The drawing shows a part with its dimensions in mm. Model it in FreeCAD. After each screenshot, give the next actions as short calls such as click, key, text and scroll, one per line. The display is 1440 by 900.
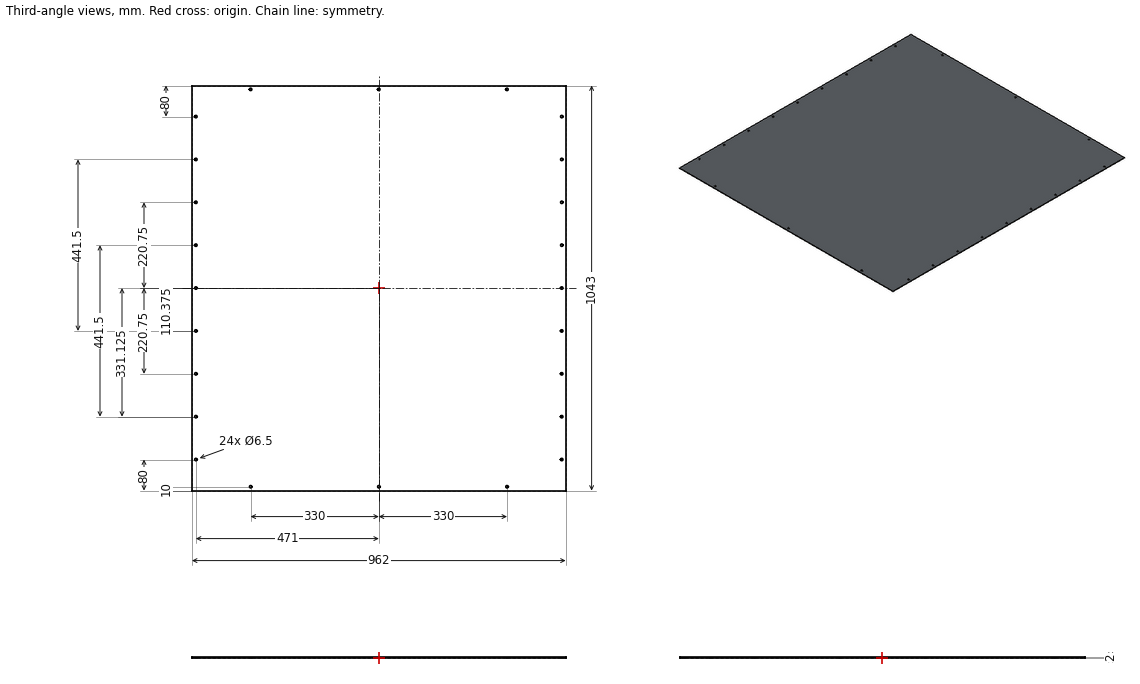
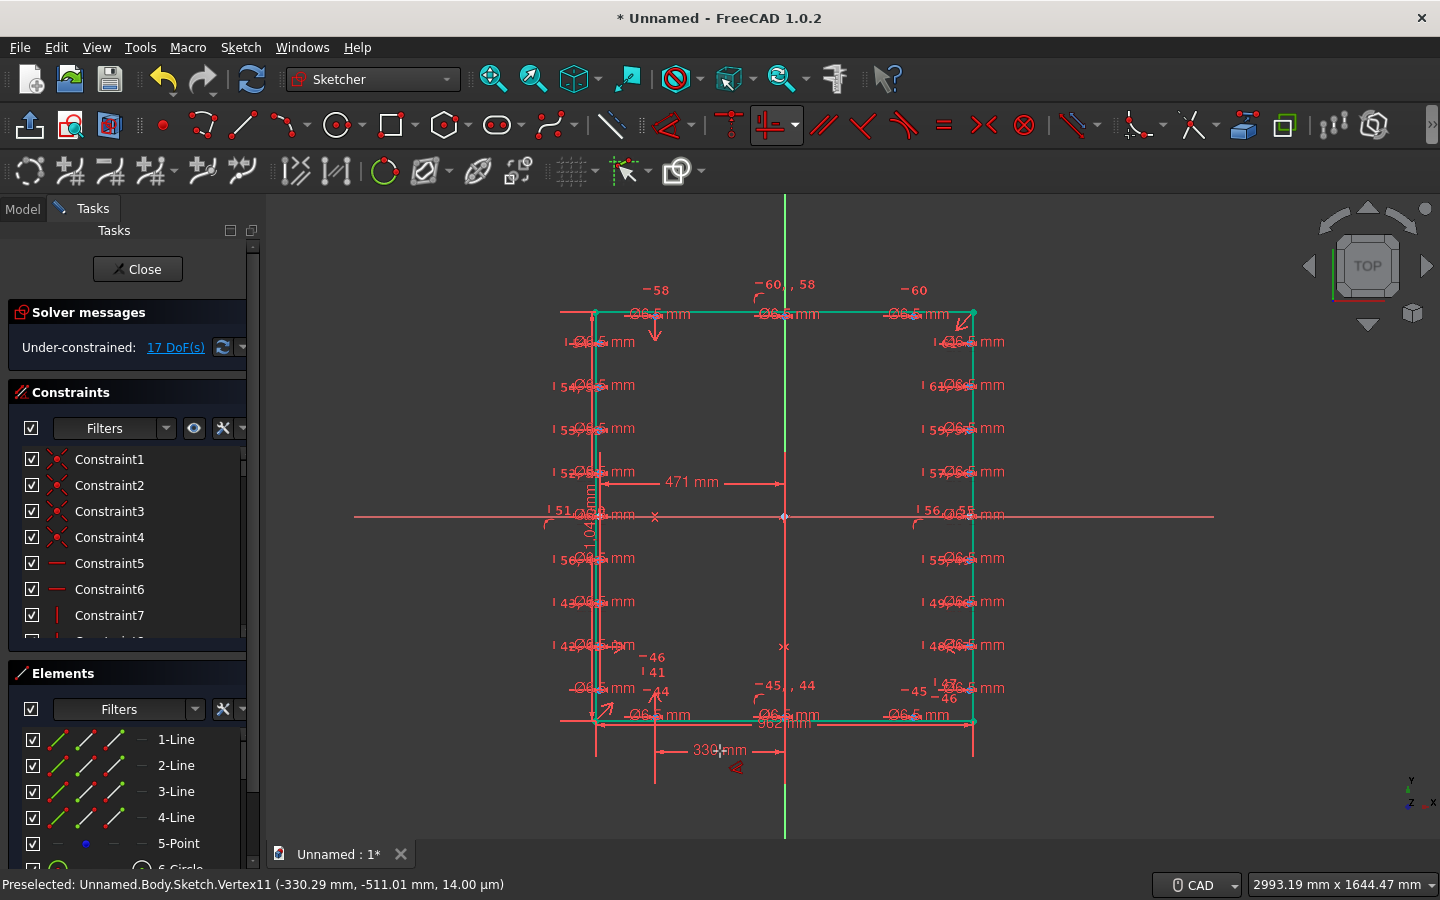
click(914, 717)
click(849, 751)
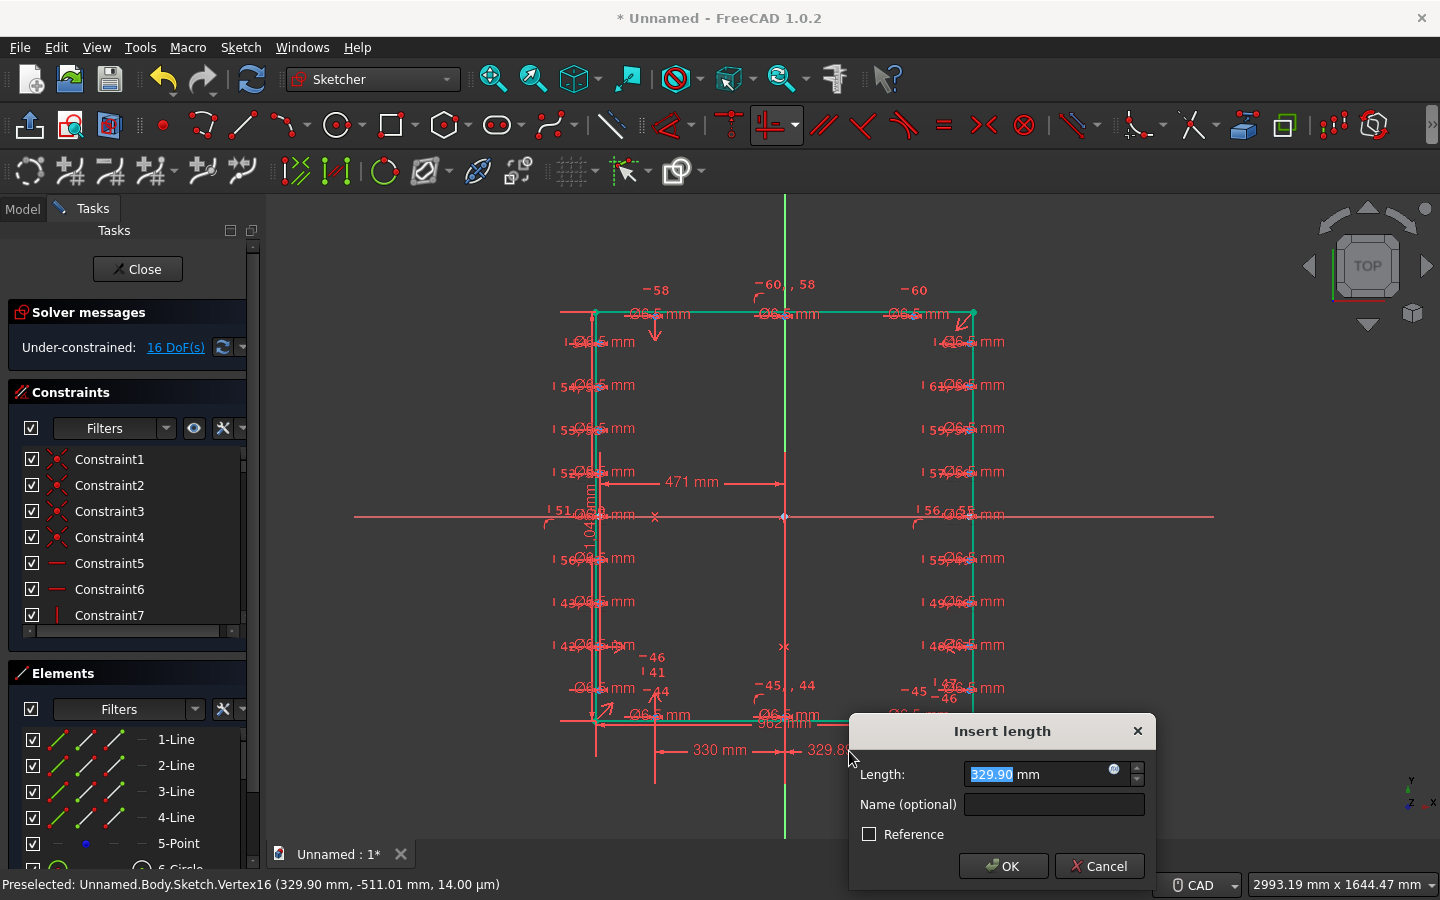
text(330)
key(Return)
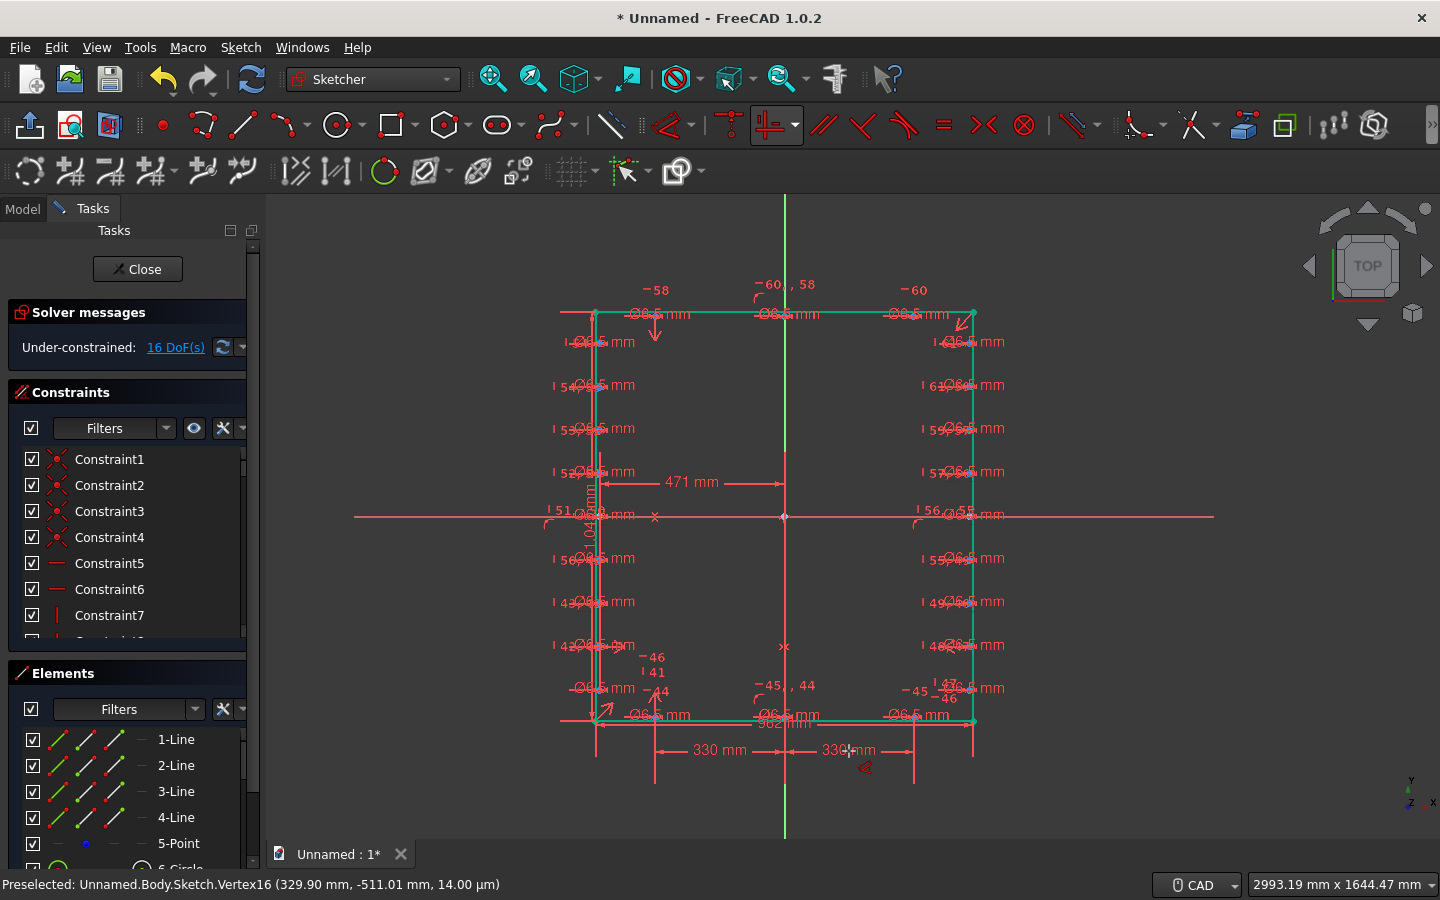
click(914, 316)
click(849, 282)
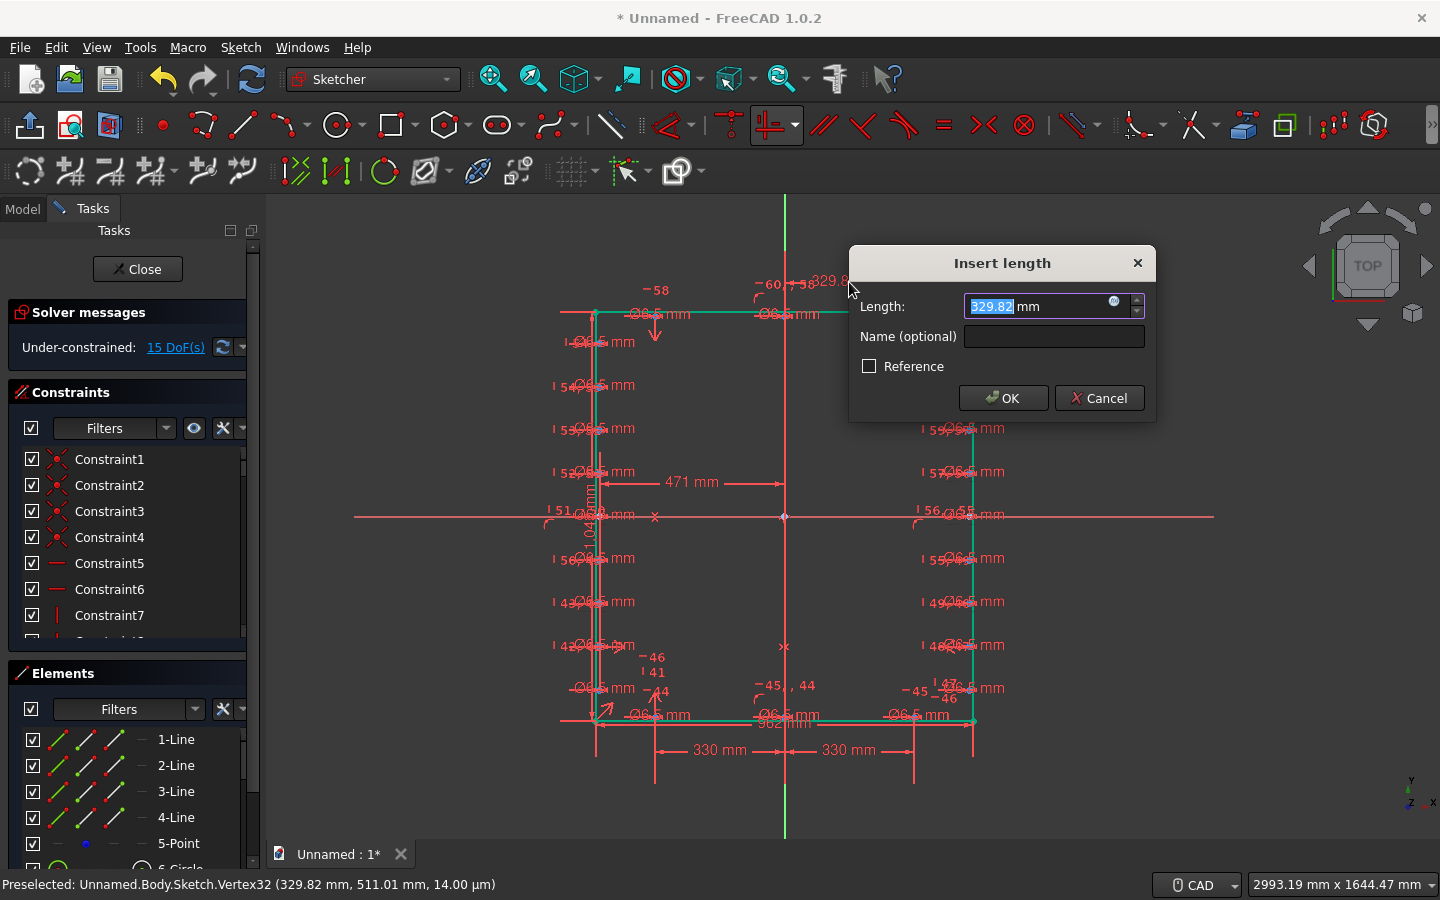
text(330)
key(Return)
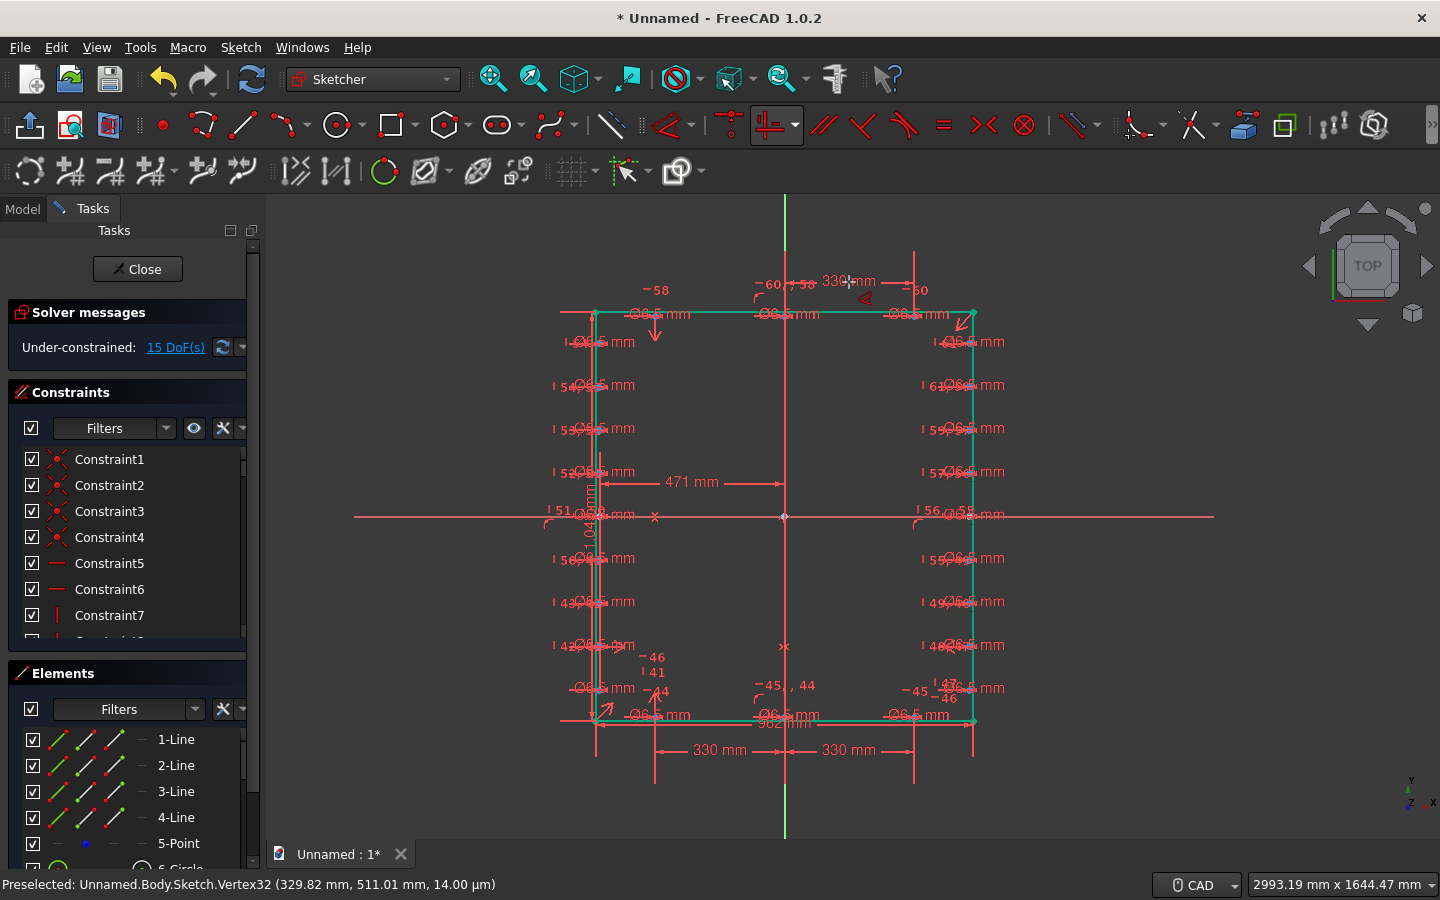
scroll(596, 721, up, 2)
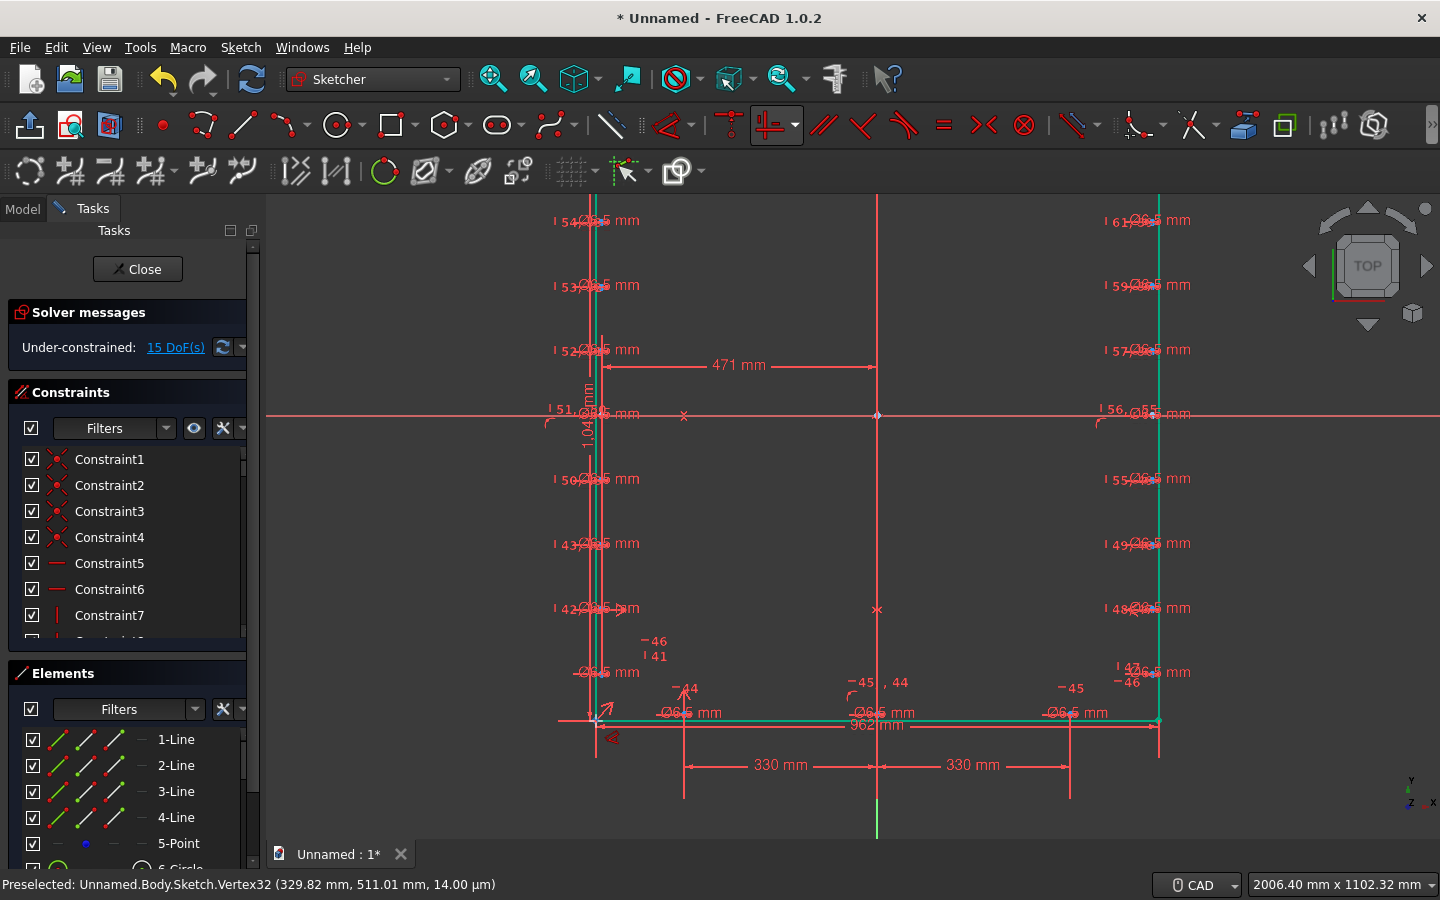
click(596, 721)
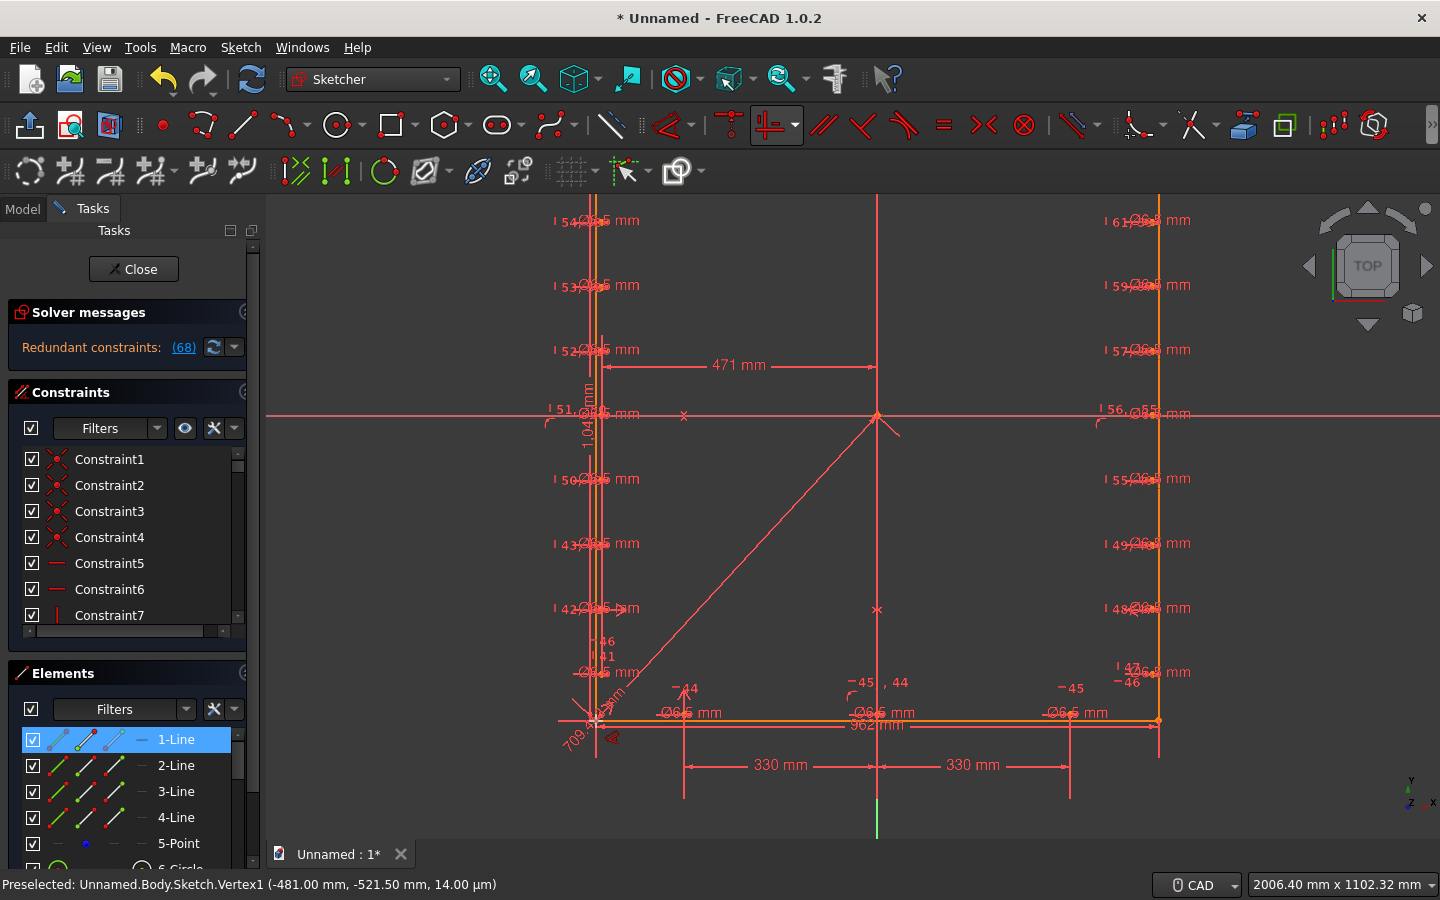
click(602, 674)
click(562, 698)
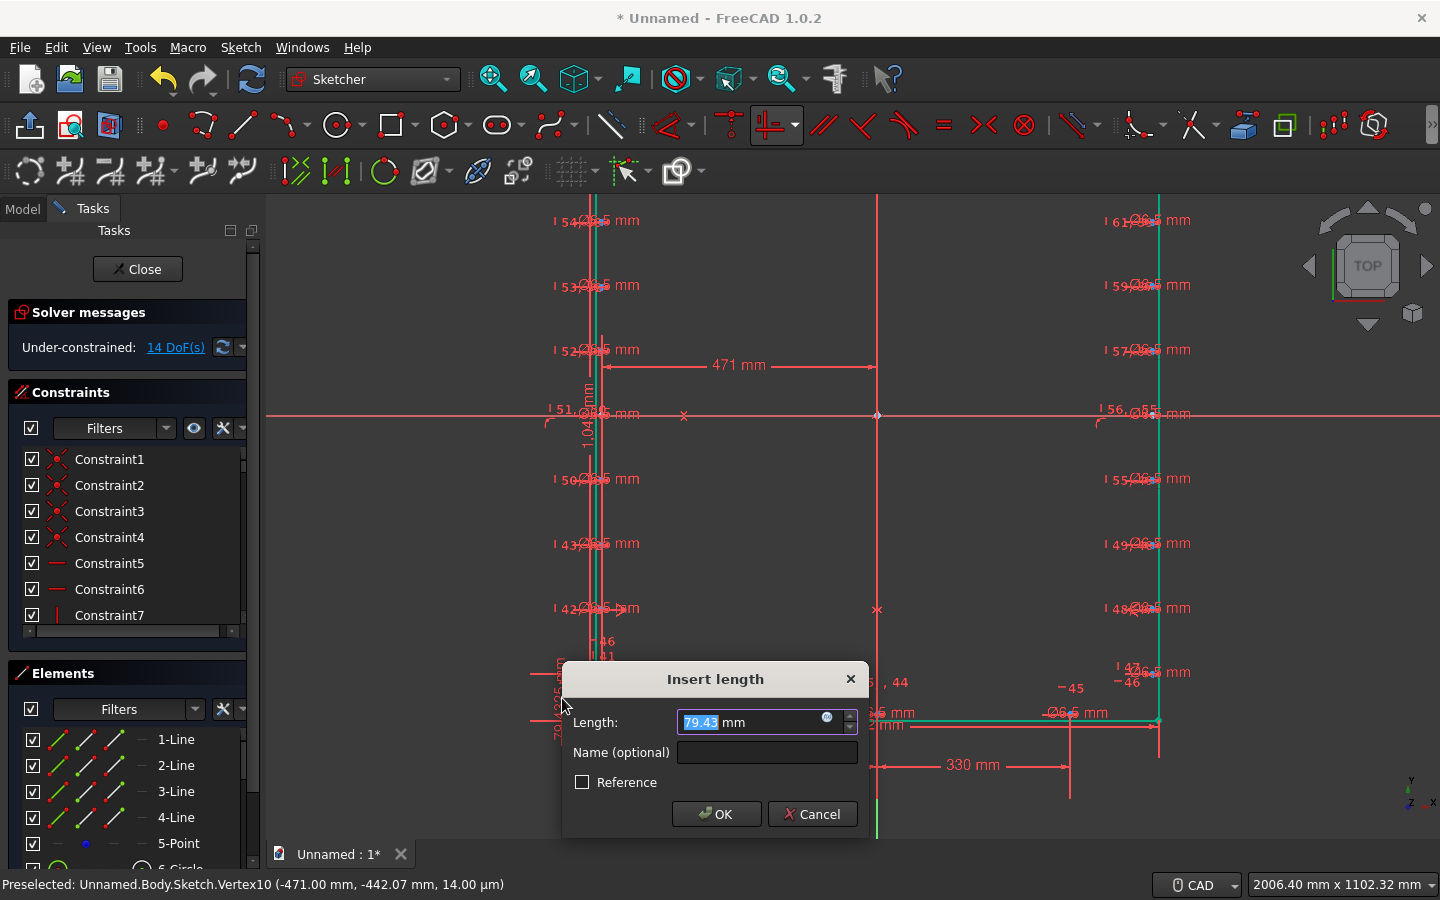
text(80)
key(Return)